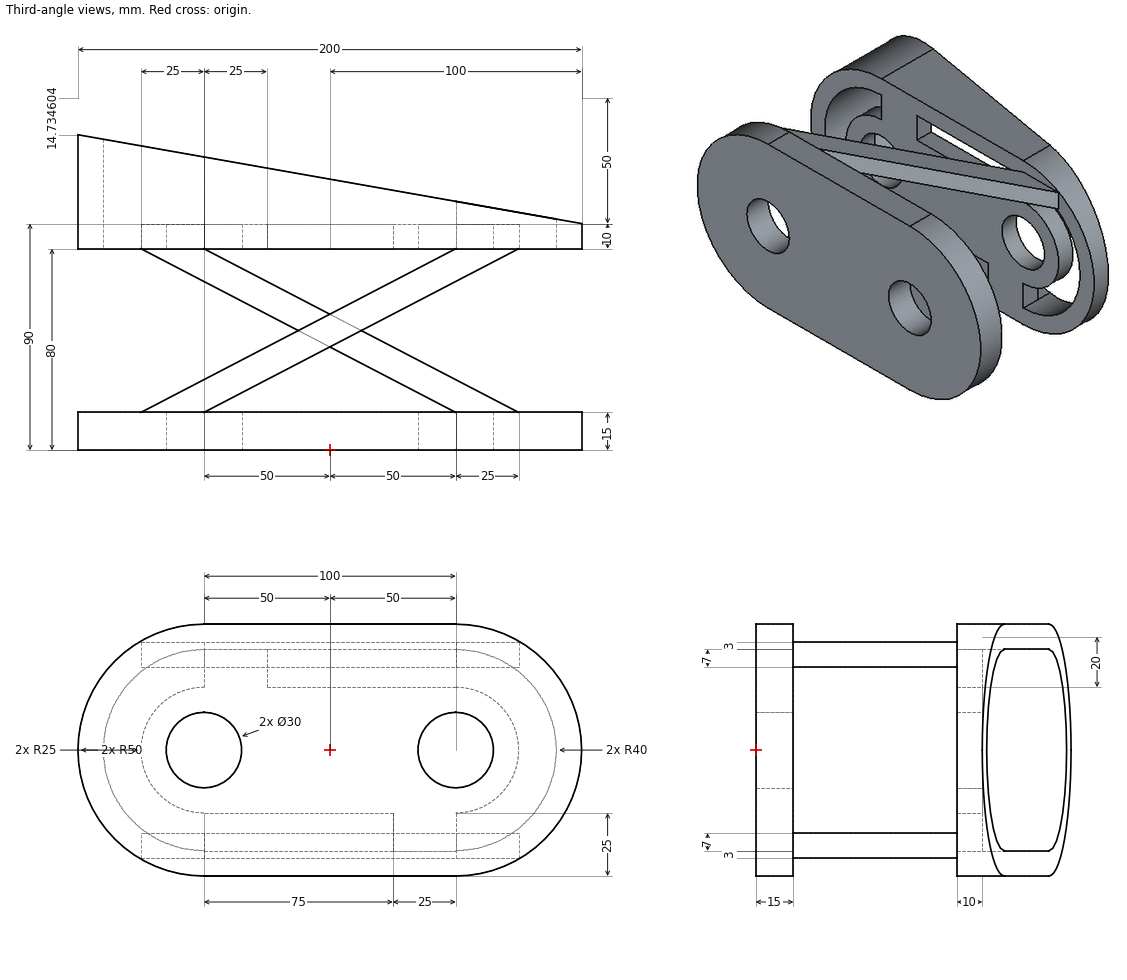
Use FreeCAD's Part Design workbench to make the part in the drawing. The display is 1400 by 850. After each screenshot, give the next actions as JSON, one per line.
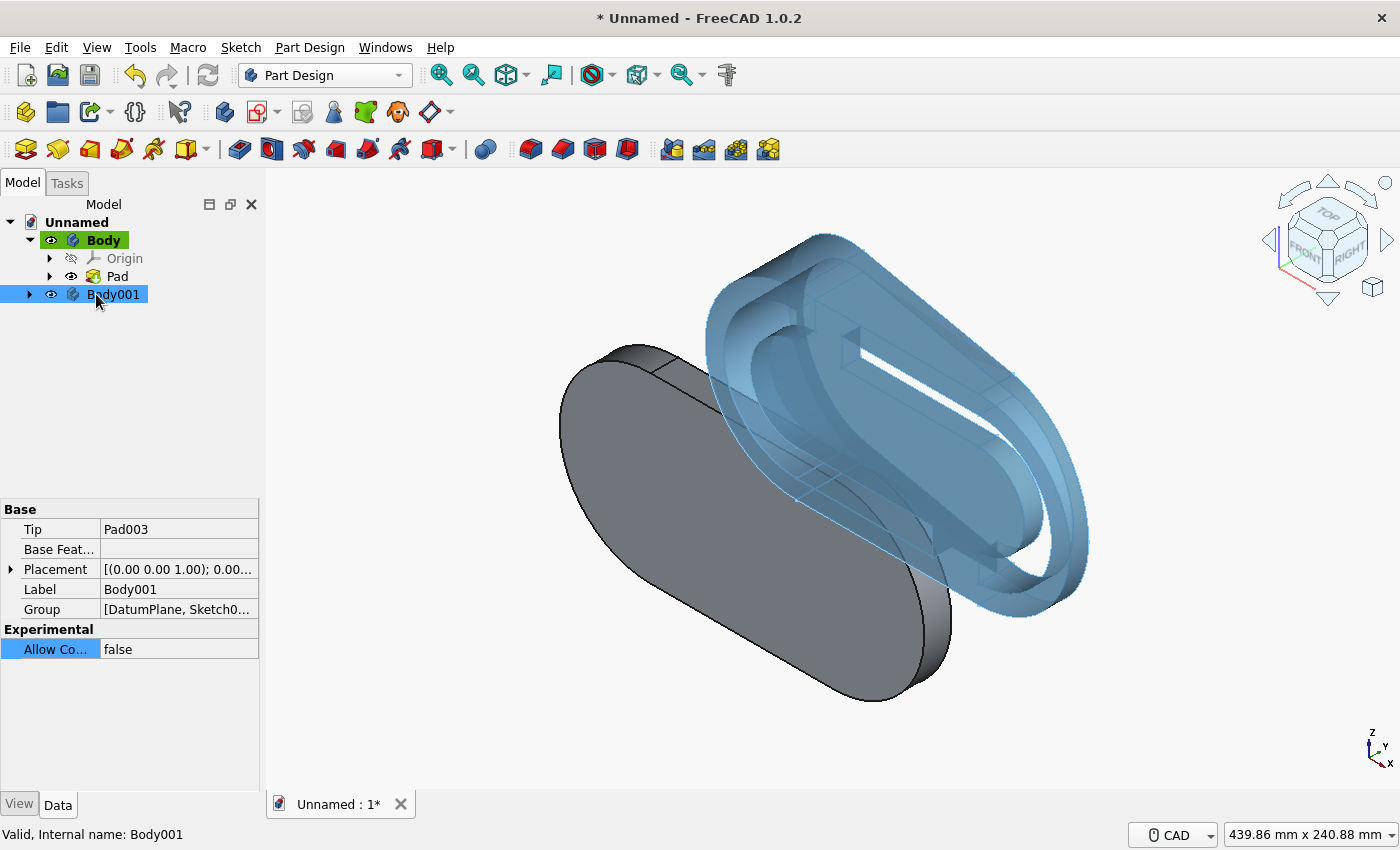
{"action": "left_click", "coordinate": [486, 150]}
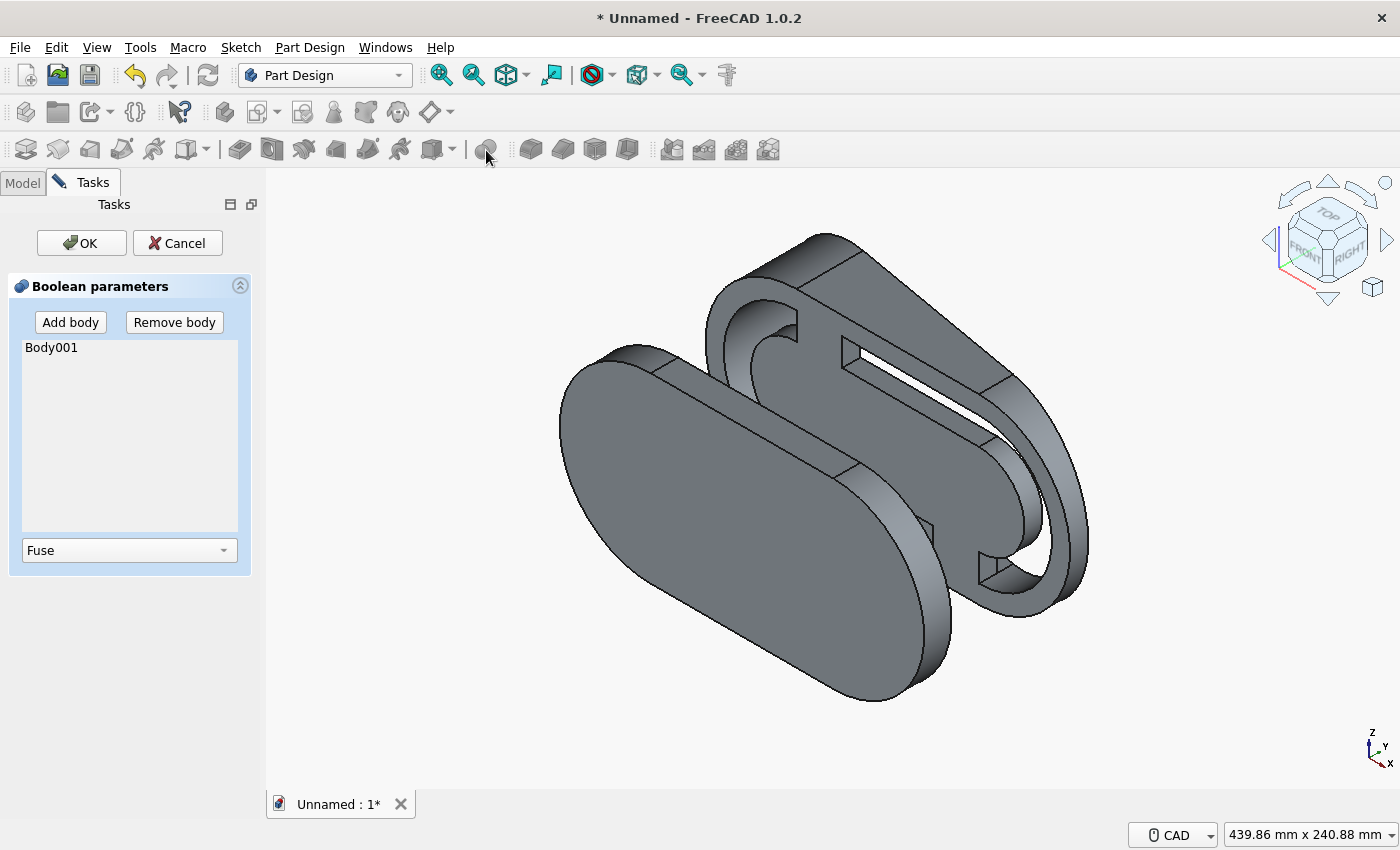
{"action": "left_click", "coordinate": [82, 243]}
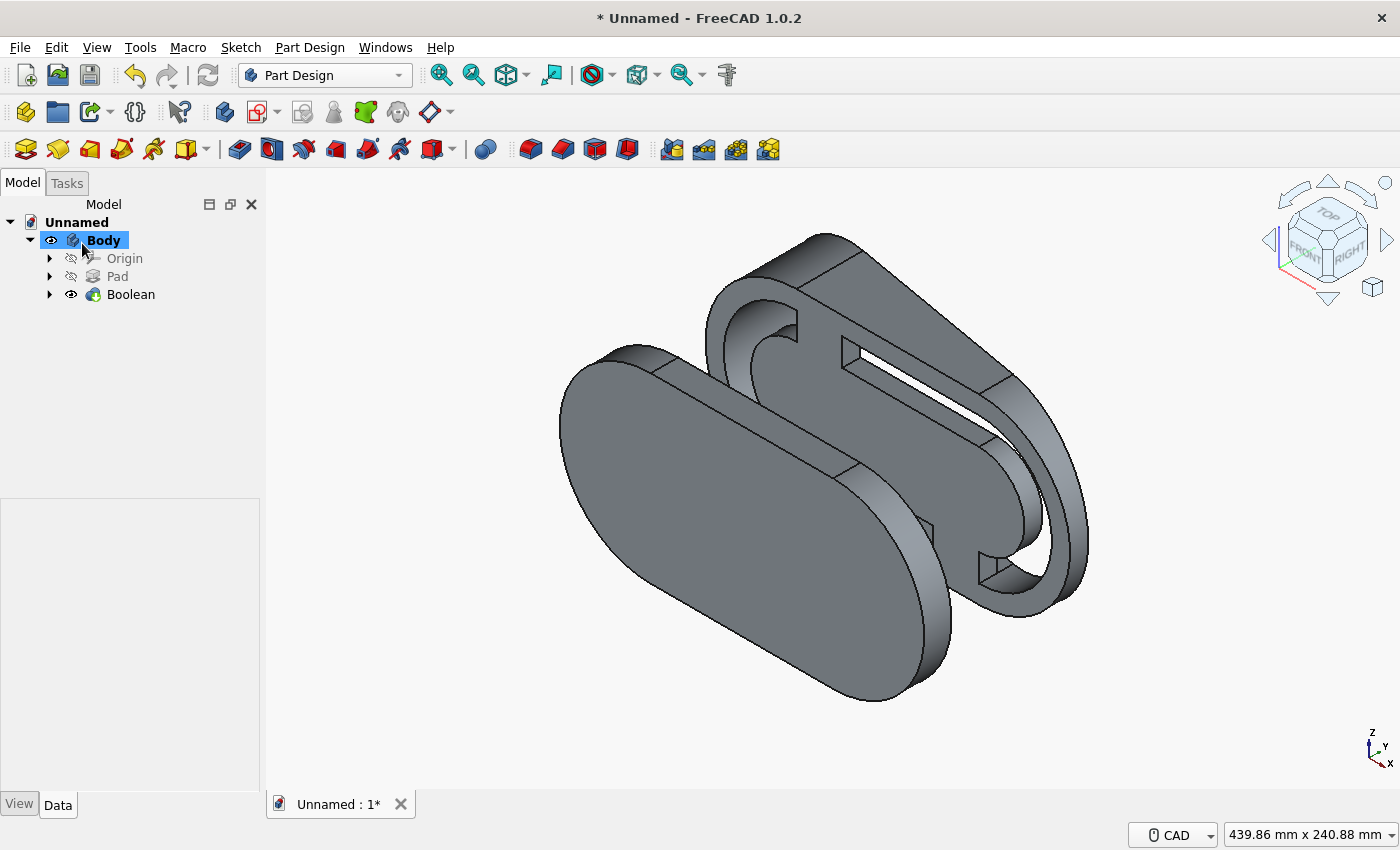
{"action": "left_click", "coordinate": [50, 258]}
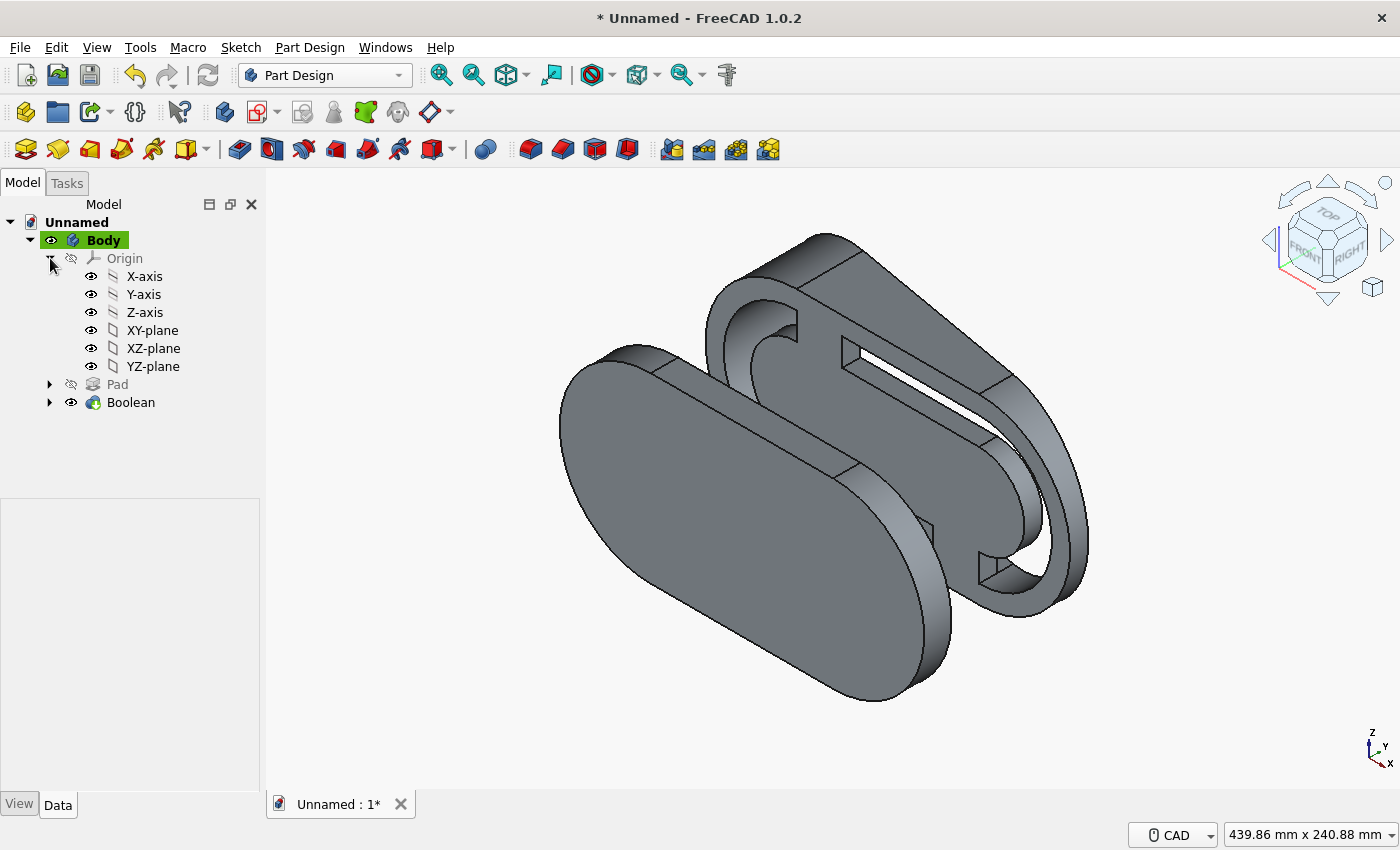
{"action": "left_click", "coordinate": [136, 330]}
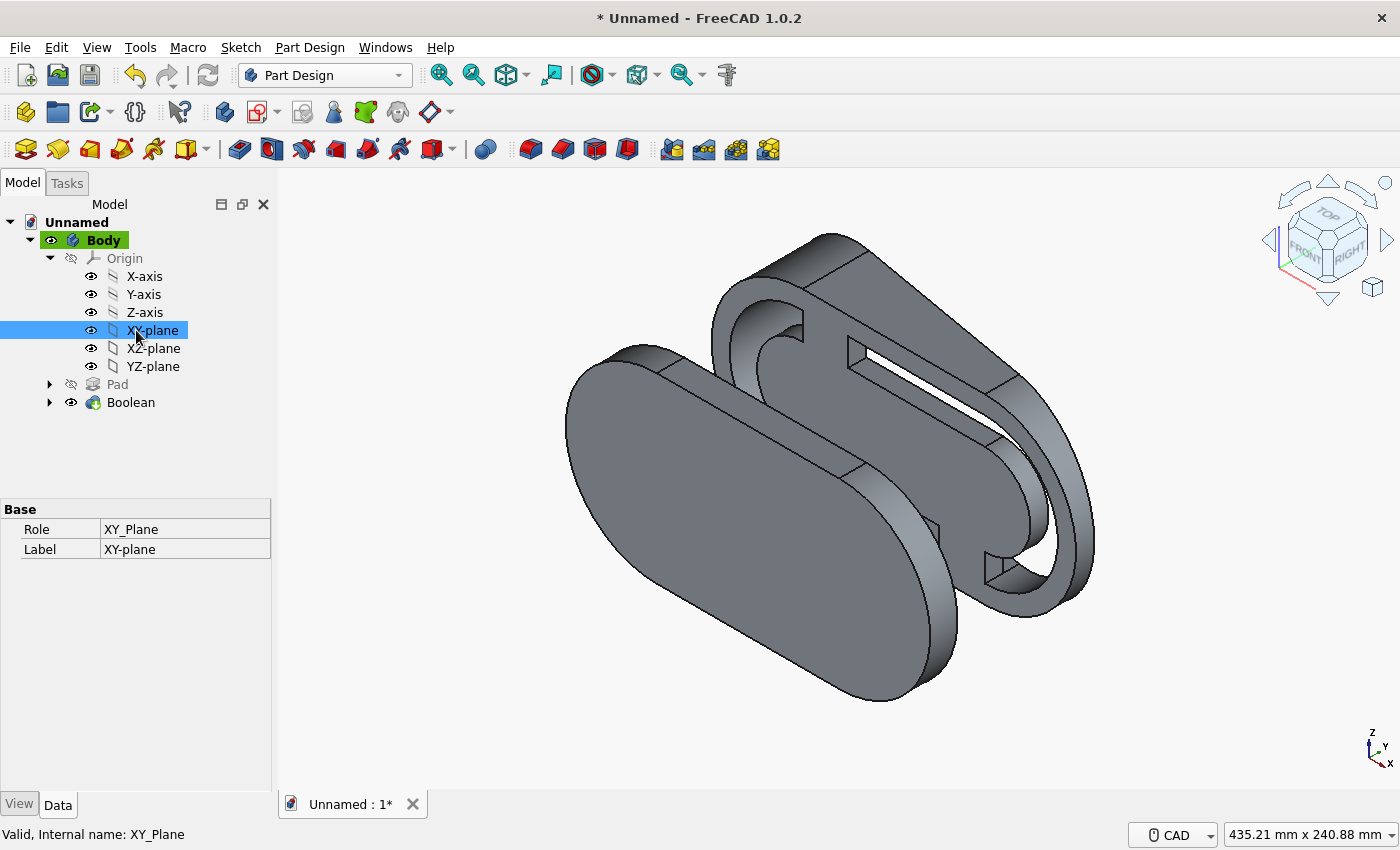
{"action": "left_click", "coordinate": [430, 112]}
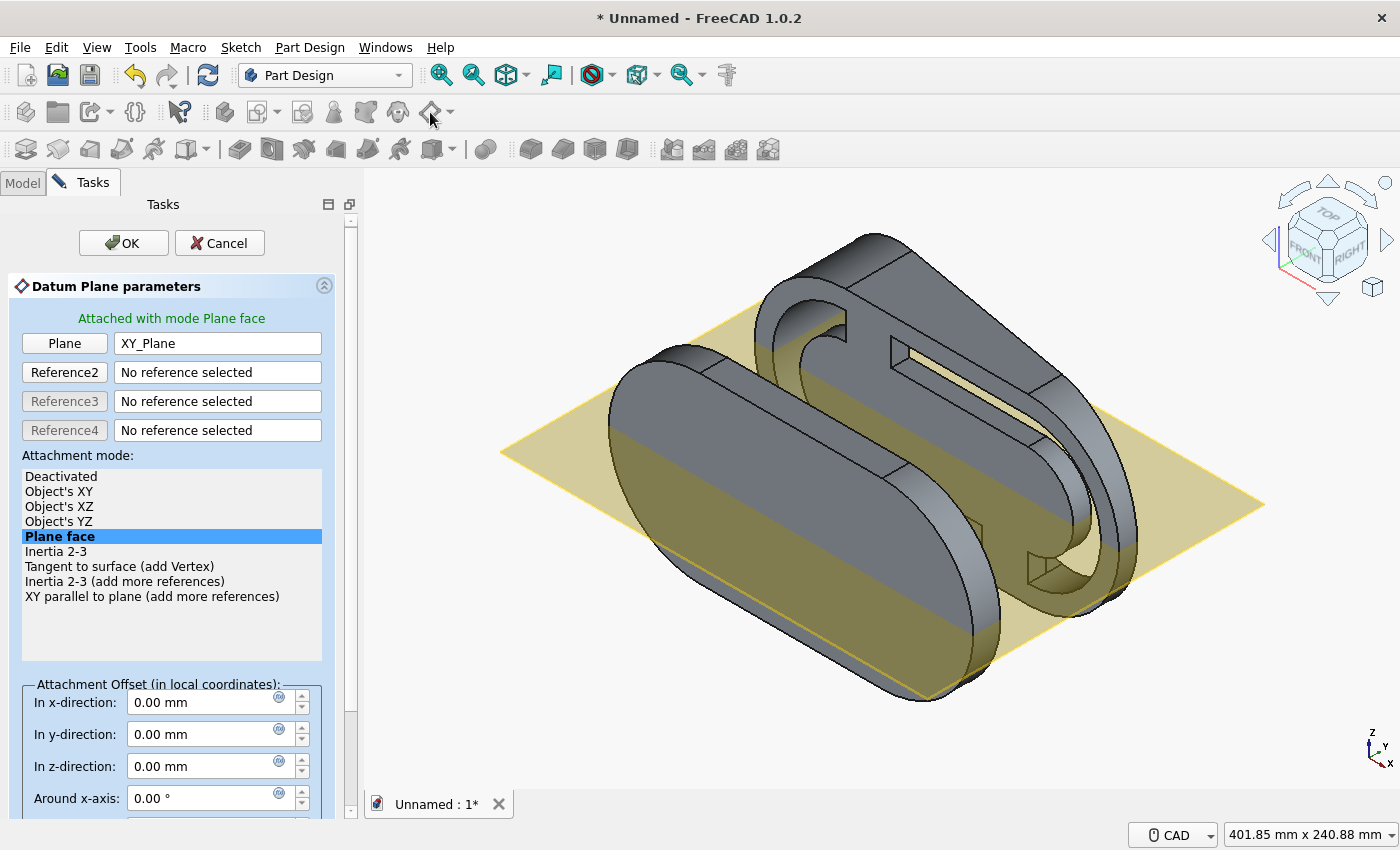
{"action": "triple_click", "coordinate": [210, 766]}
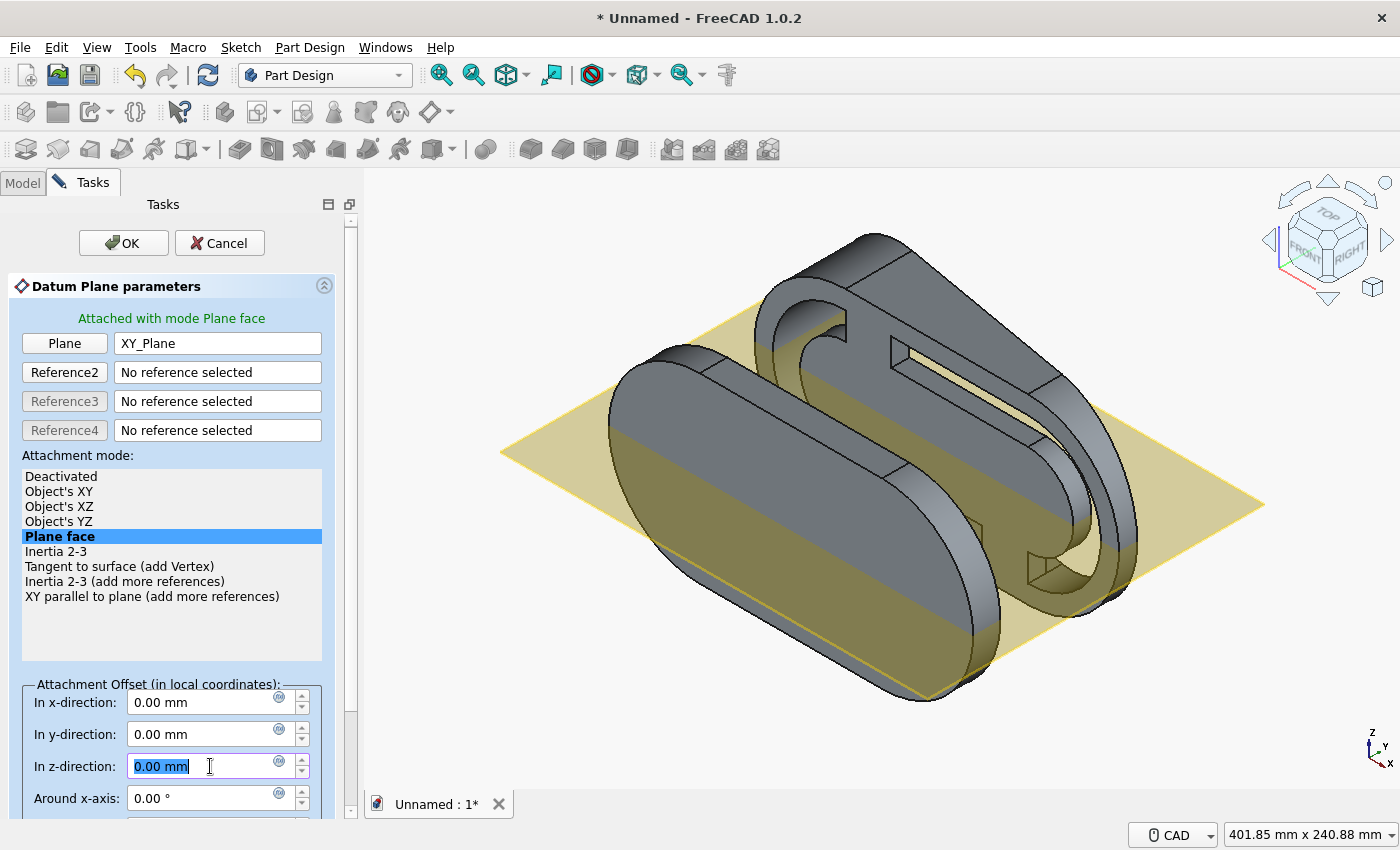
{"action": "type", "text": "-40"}
{"action": "key", "text": "Tab"}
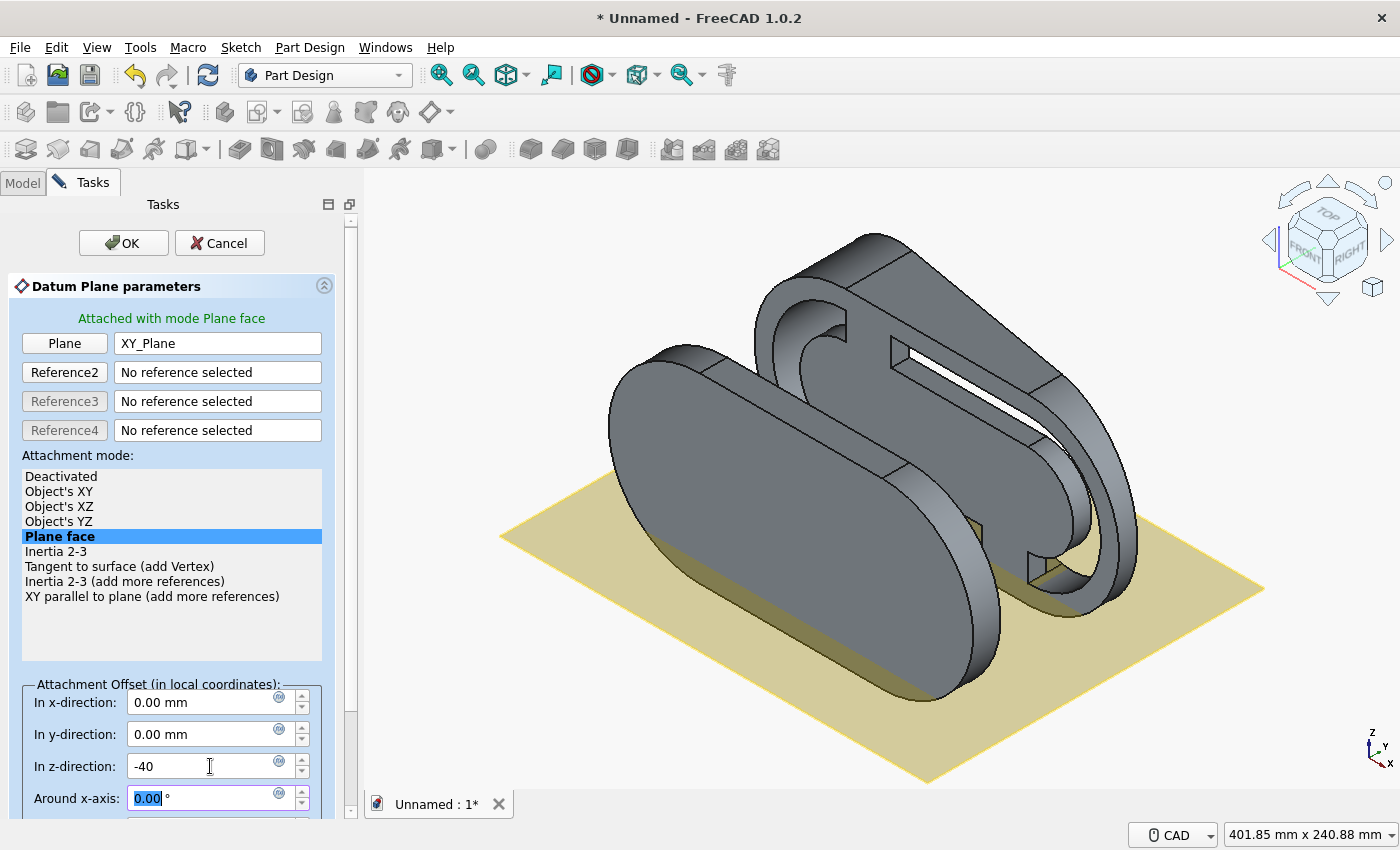
{"action": "left_click", "coordinate": [124, 243]}